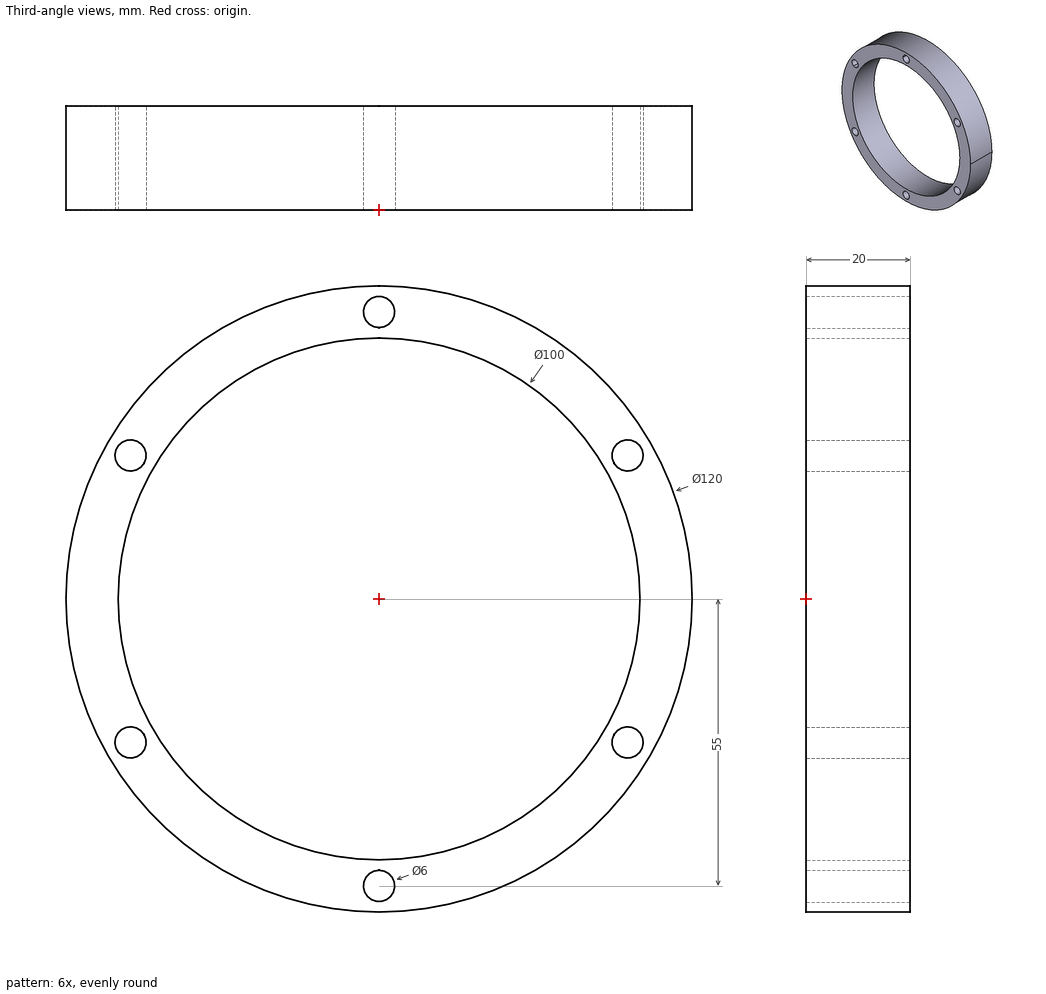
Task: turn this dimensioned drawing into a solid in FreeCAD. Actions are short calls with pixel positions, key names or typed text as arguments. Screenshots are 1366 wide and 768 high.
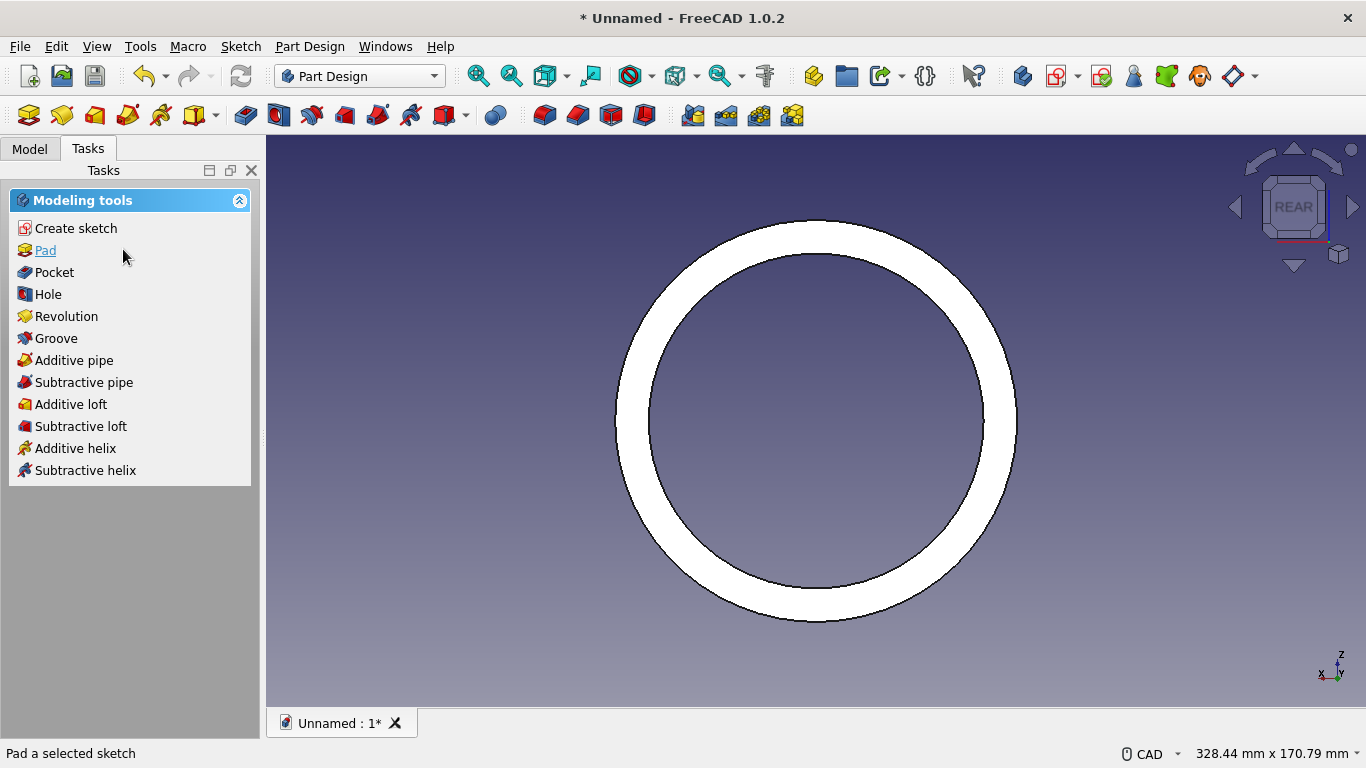
click(246, 116)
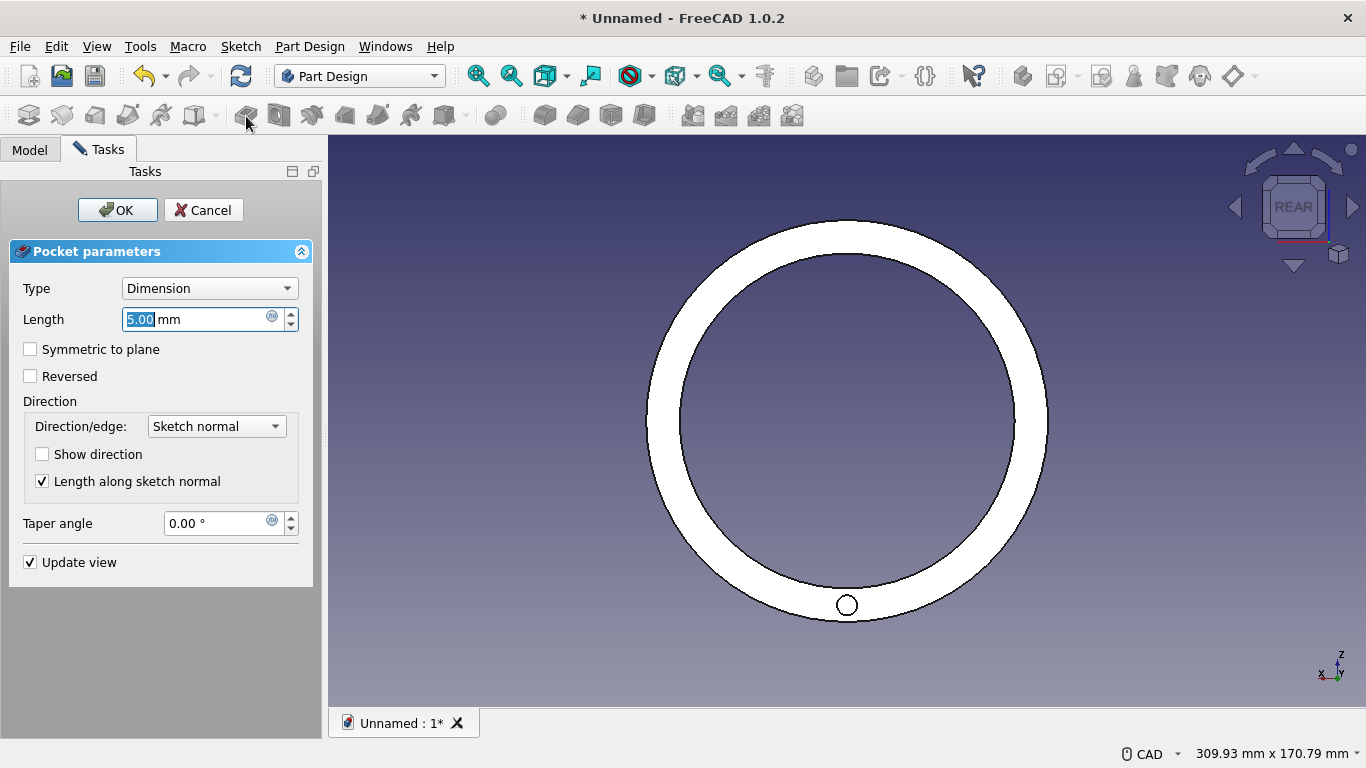
click(210, 288)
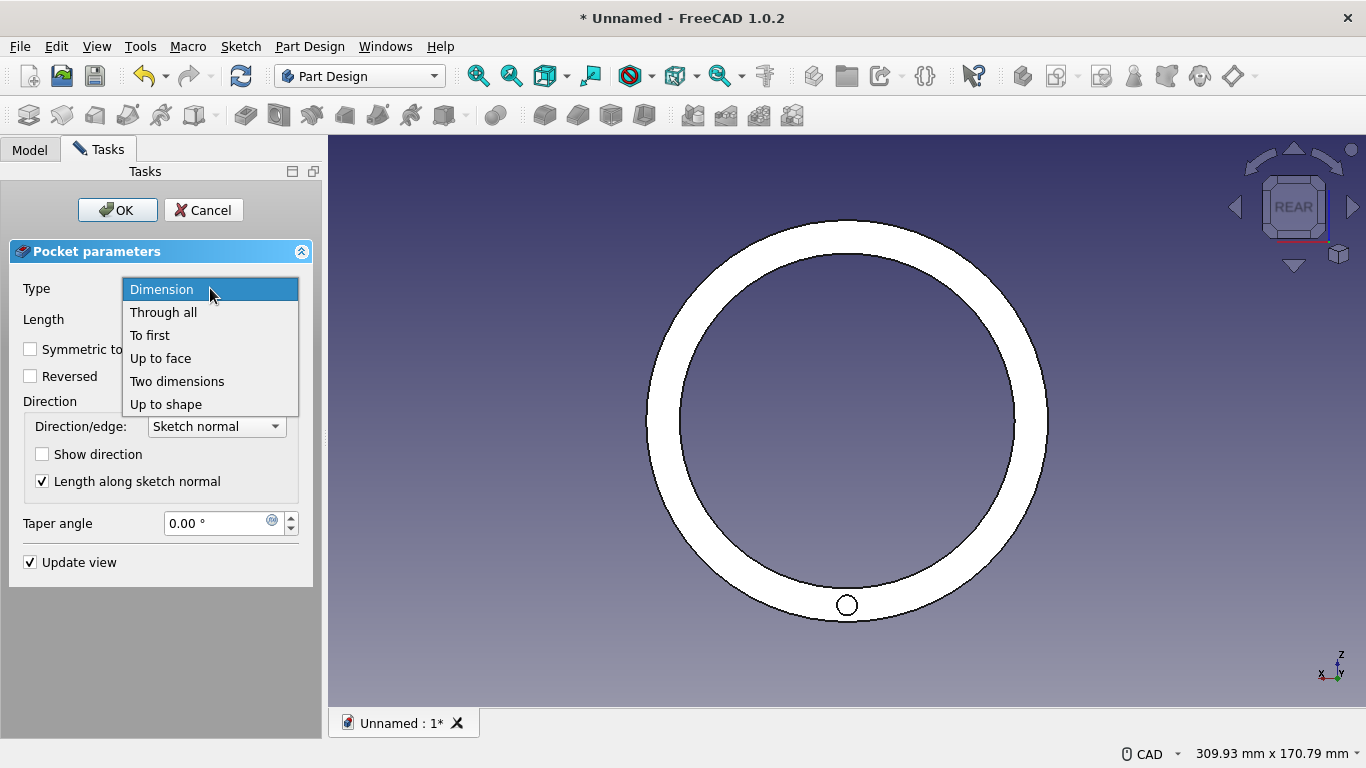
click(208, 312)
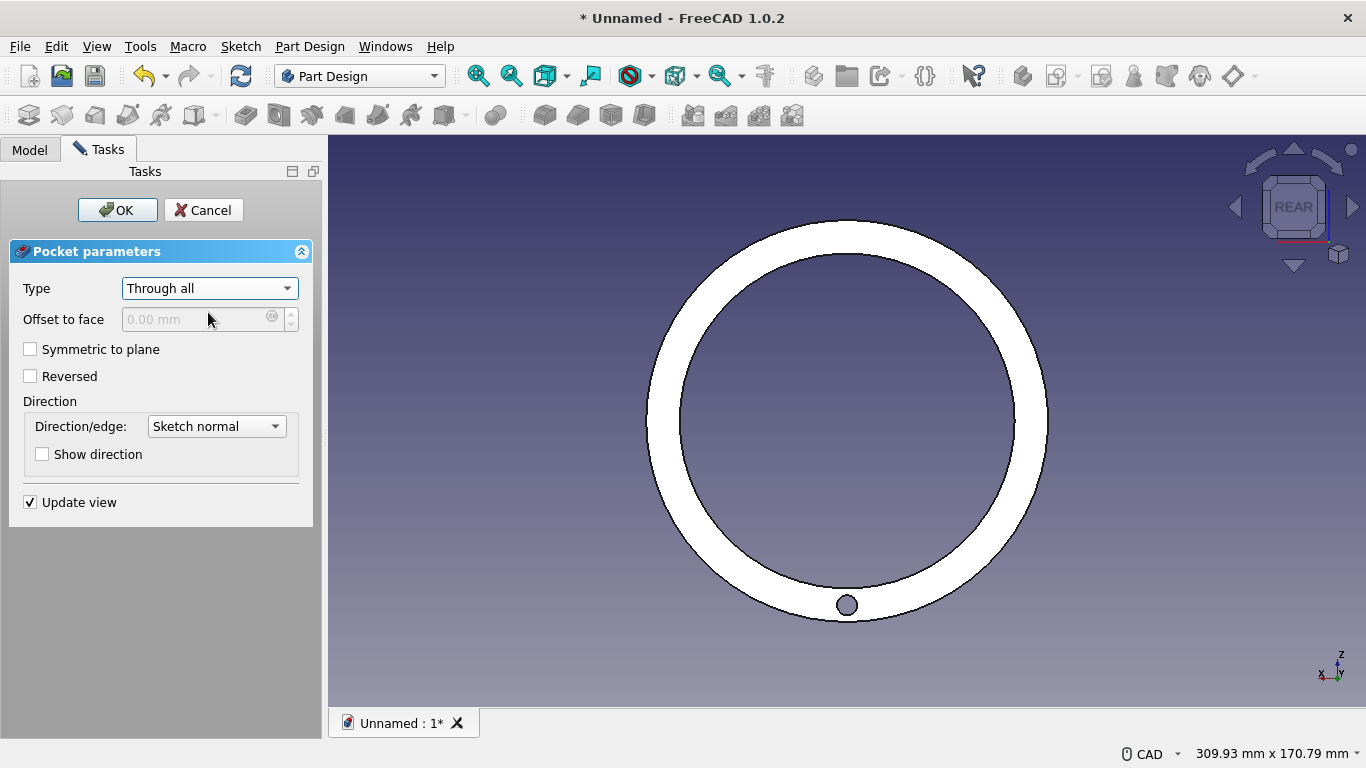
click(118, 210)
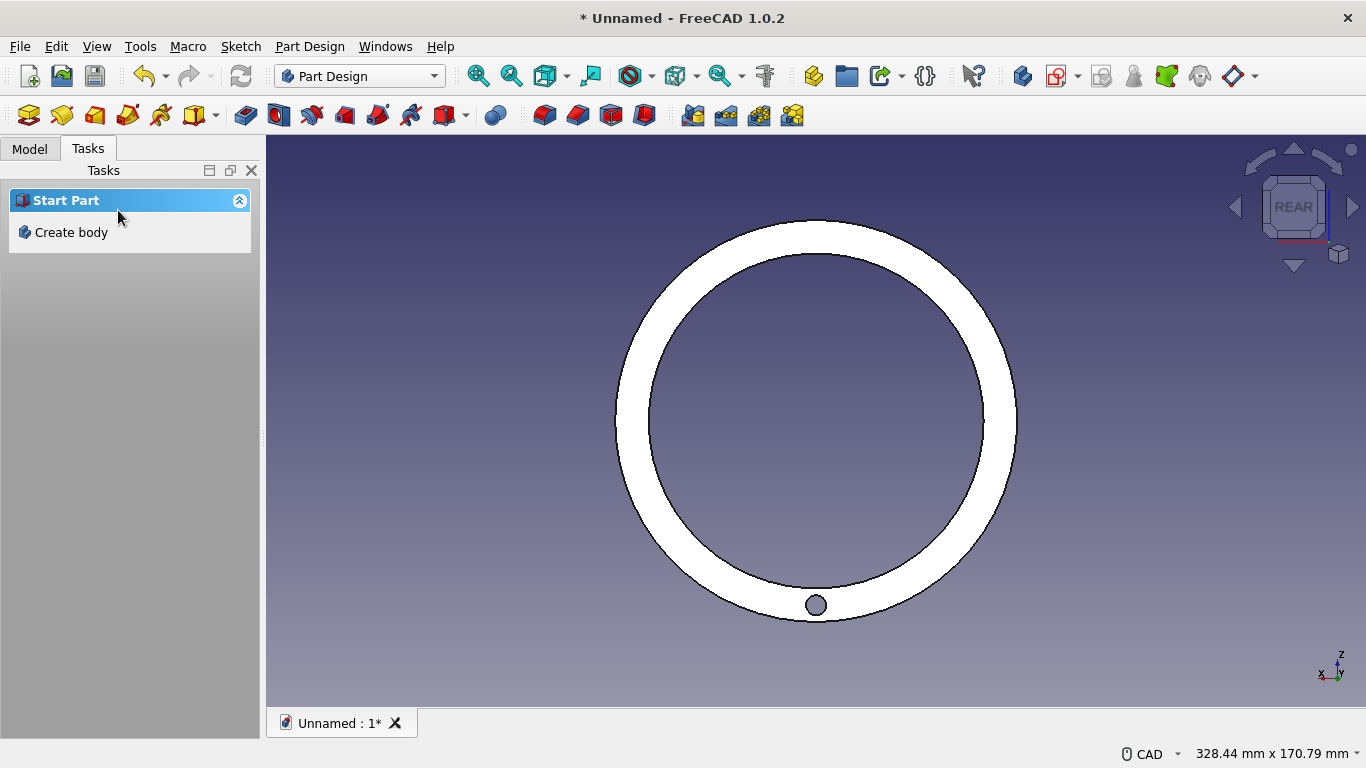
click(30, 148)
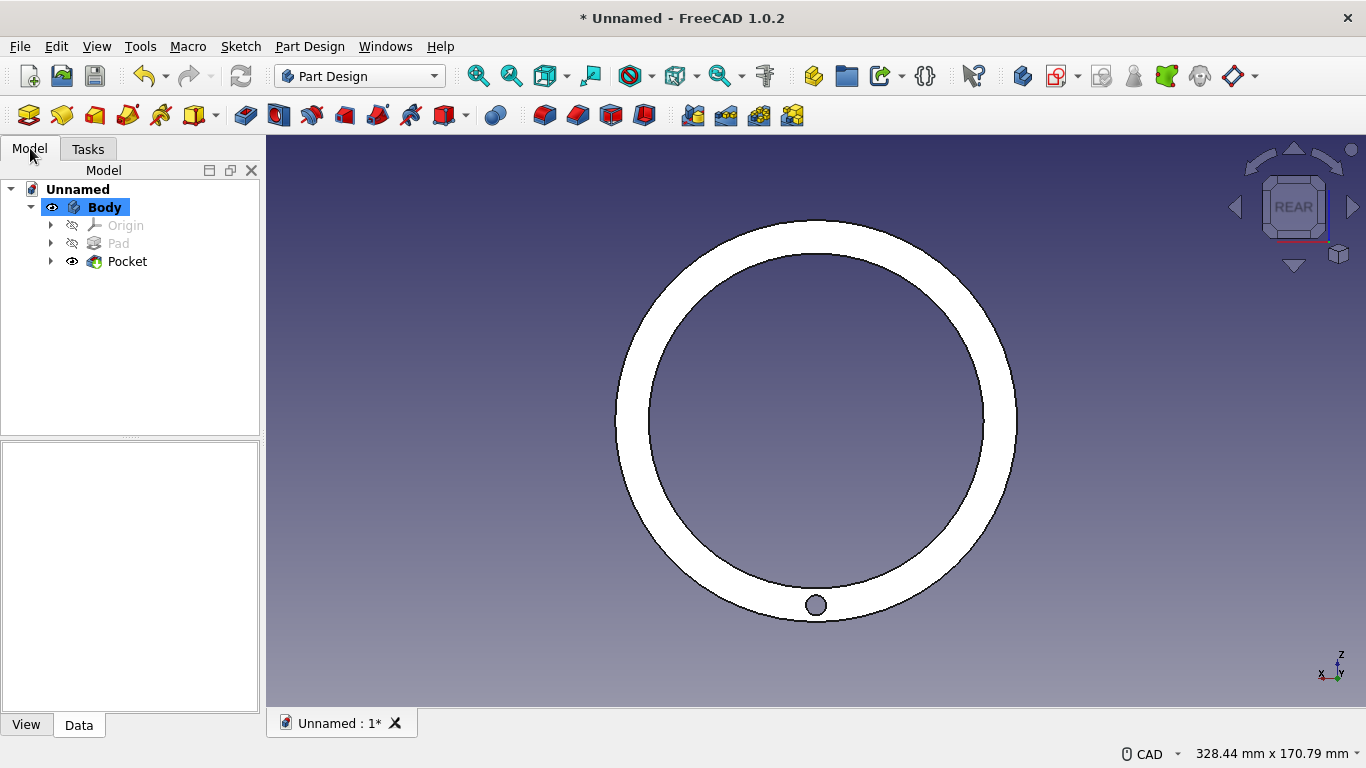
click(117, 261)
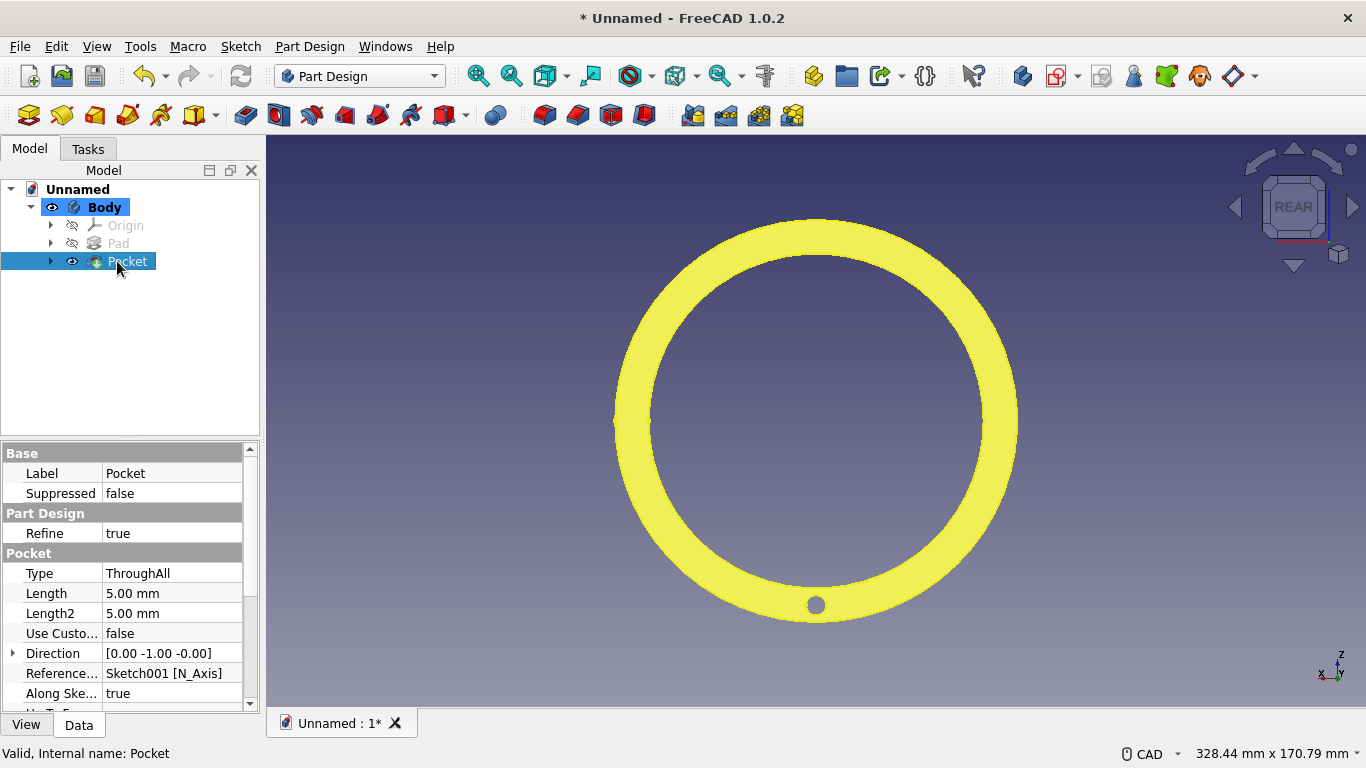
click(759, 116)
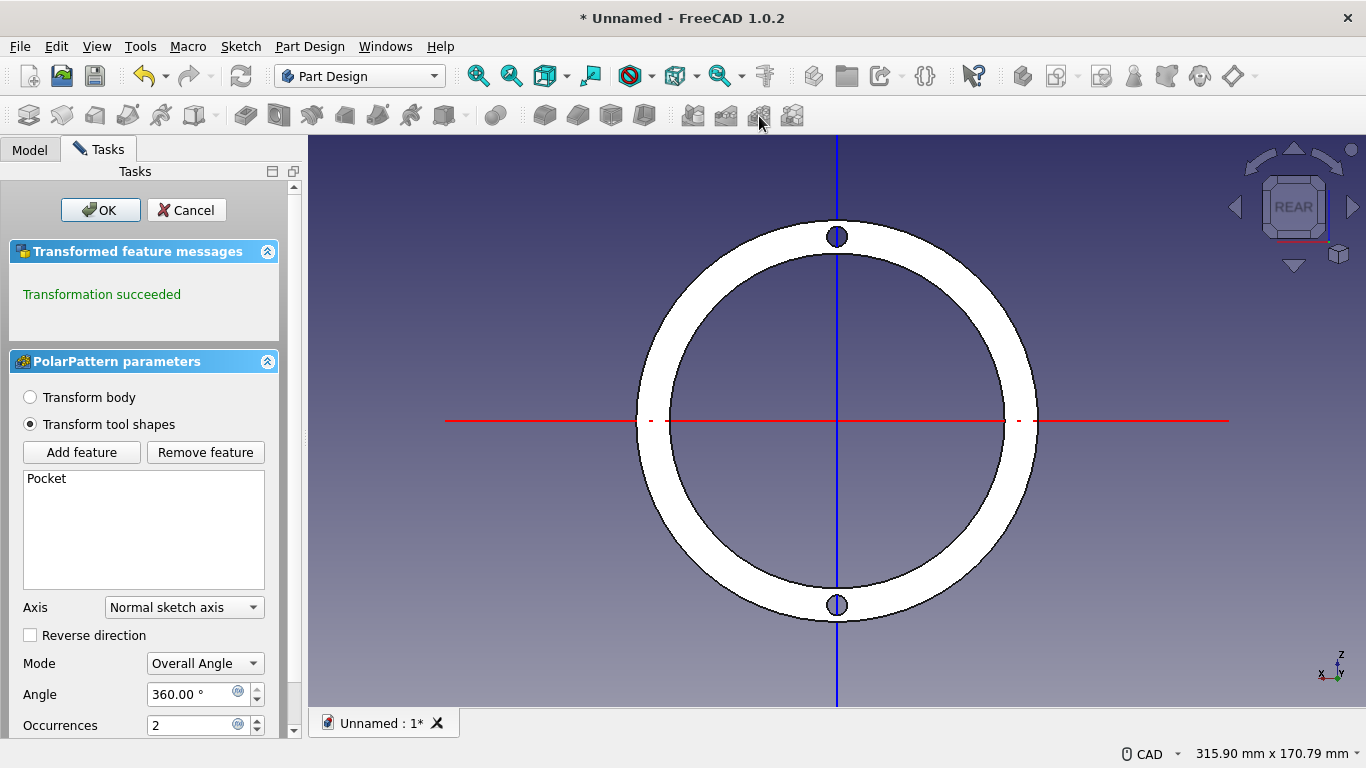
click(185, 608)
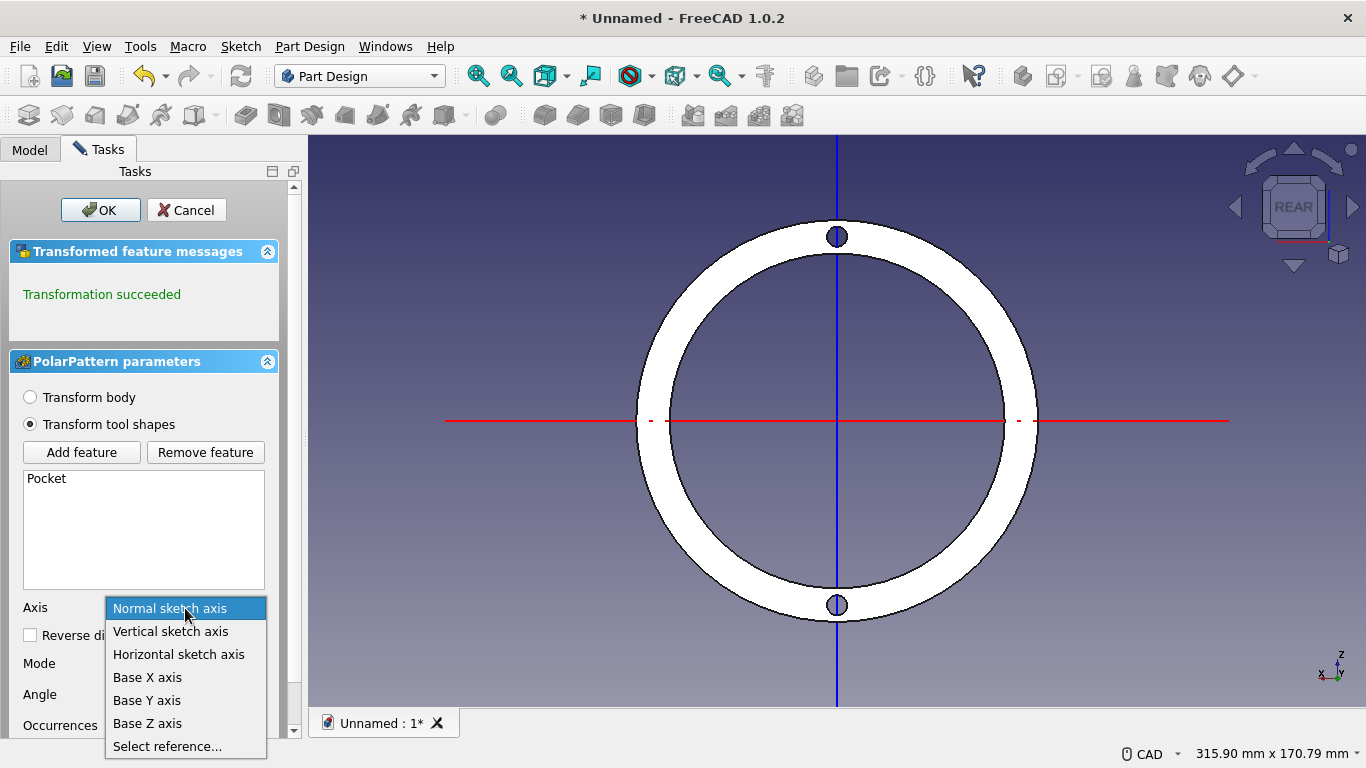
click(184, 700)